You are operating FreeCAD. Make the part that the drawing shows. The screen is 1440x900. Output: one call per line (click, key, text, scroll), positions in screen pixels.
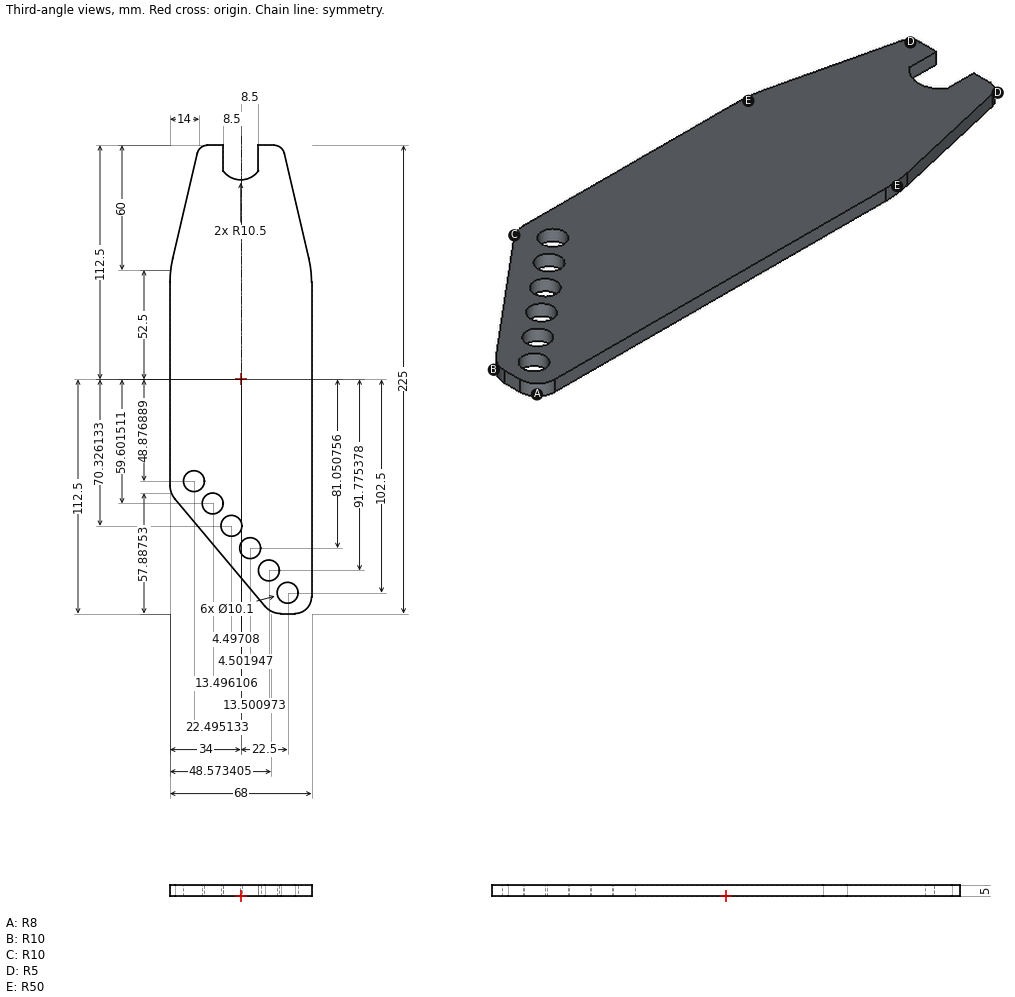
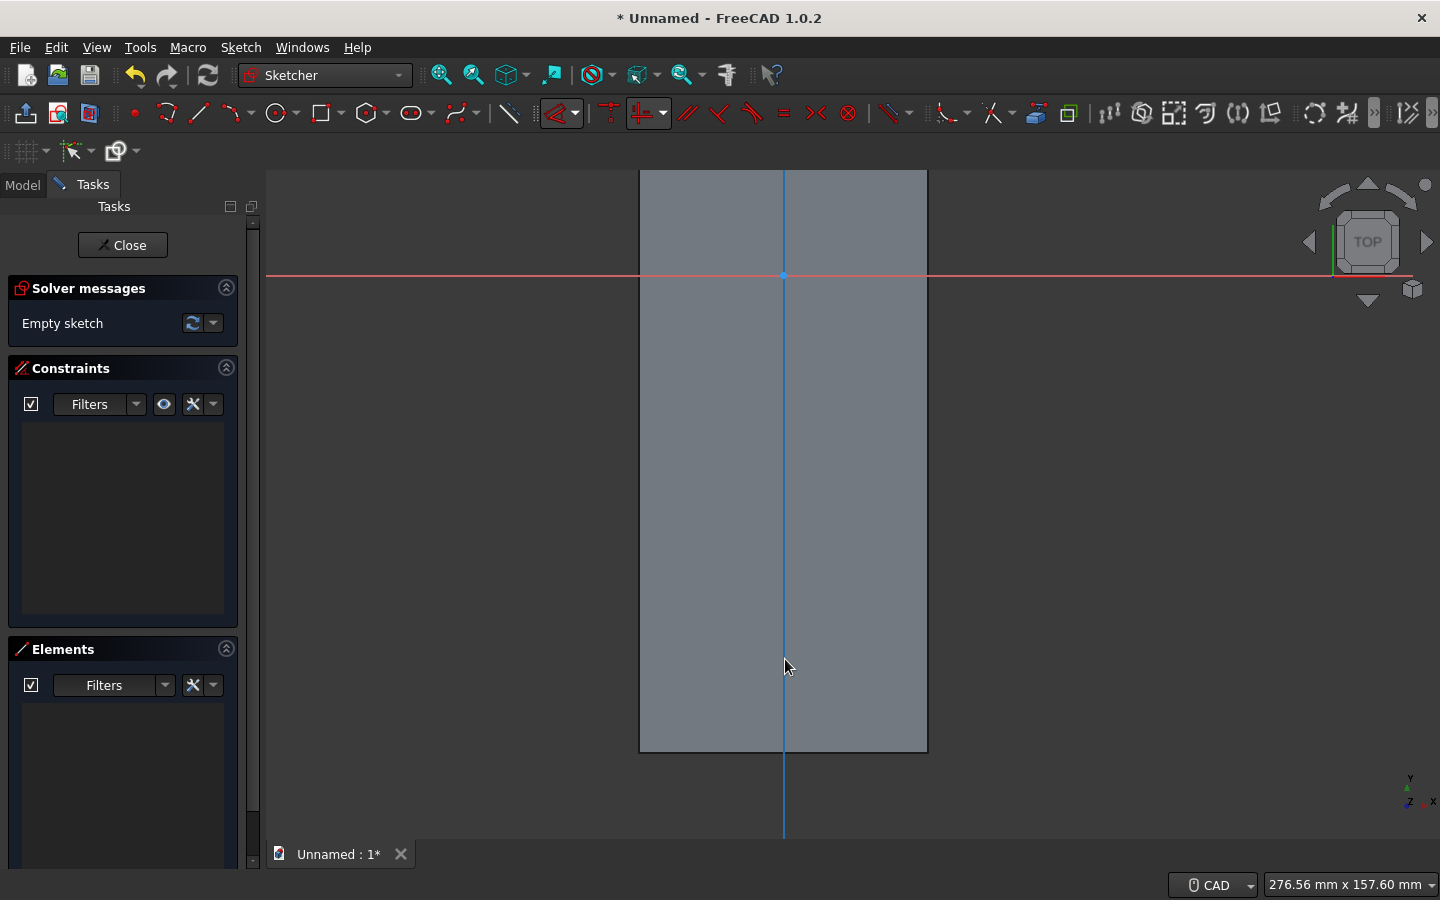
key(g)
key(c)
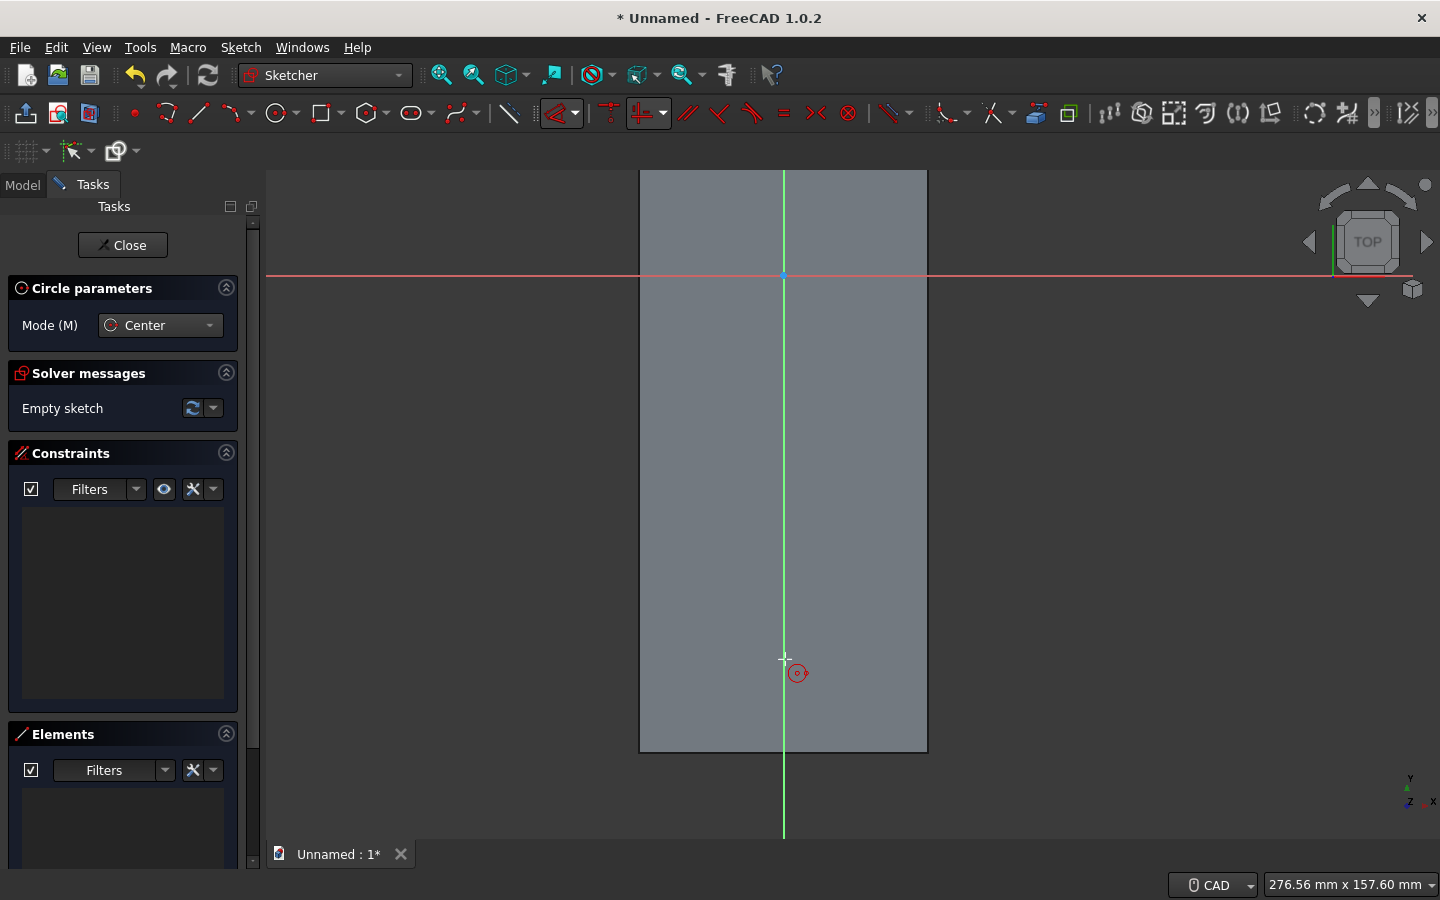
click(879, 711)
click(894, 696)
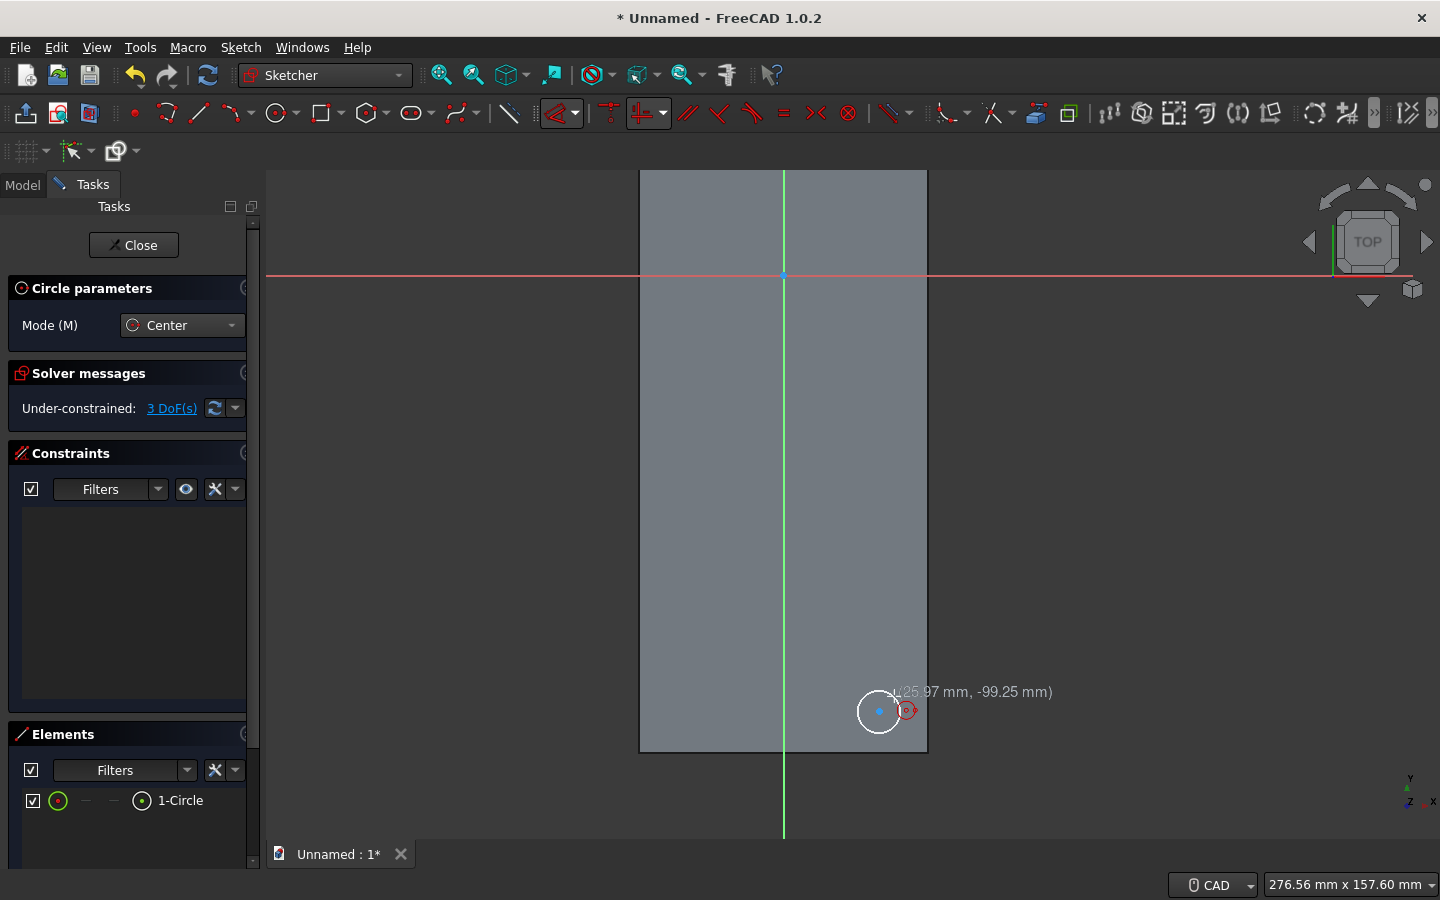
click(841, 665)
click(856, 650)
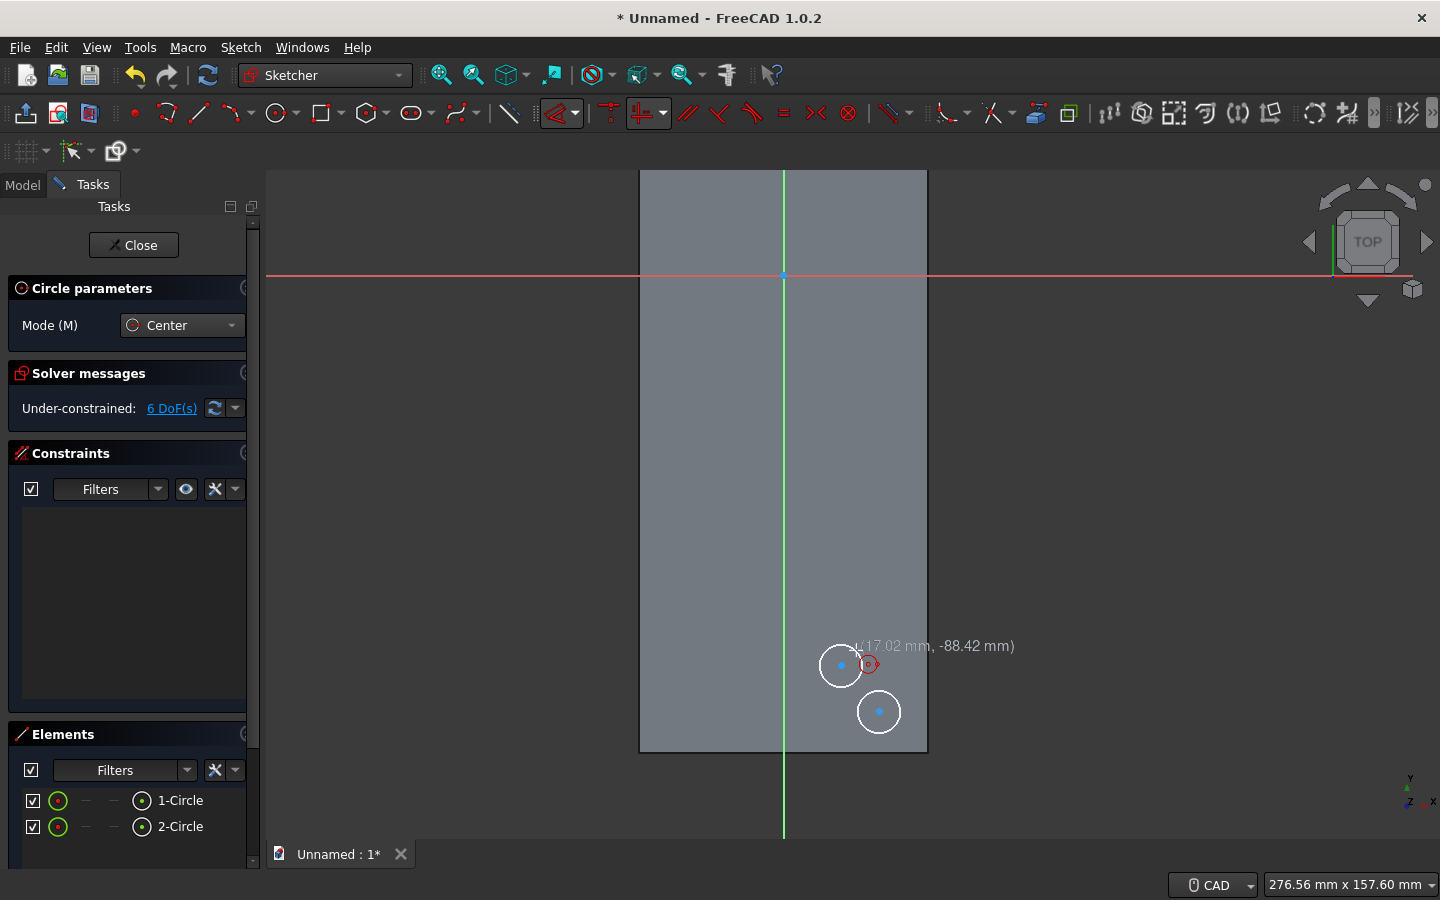
click(803, 620)
click(818, 605)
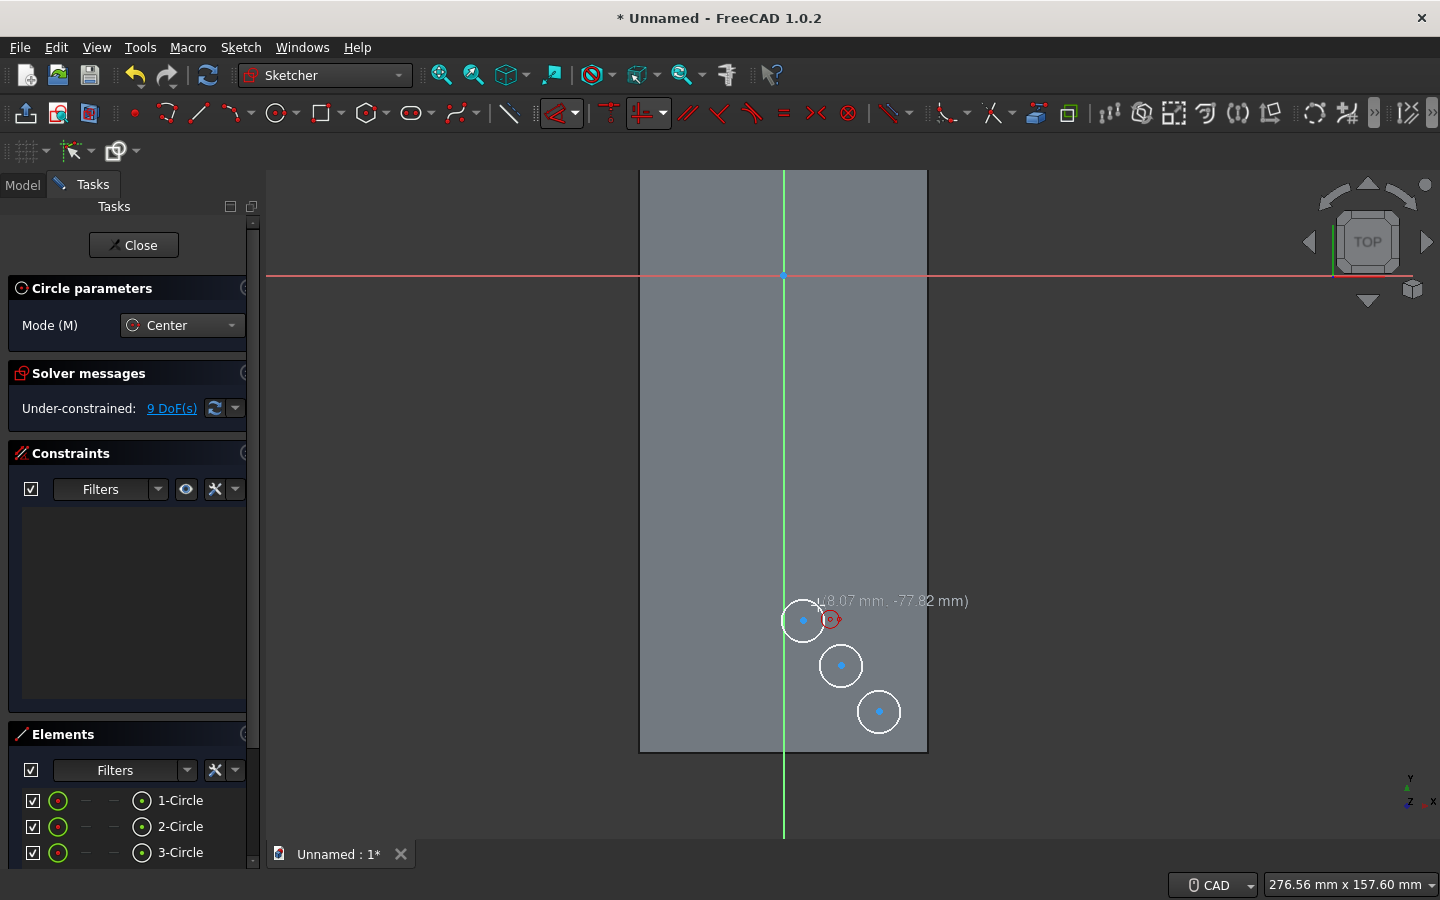
click(765, 574)
click(749, 559)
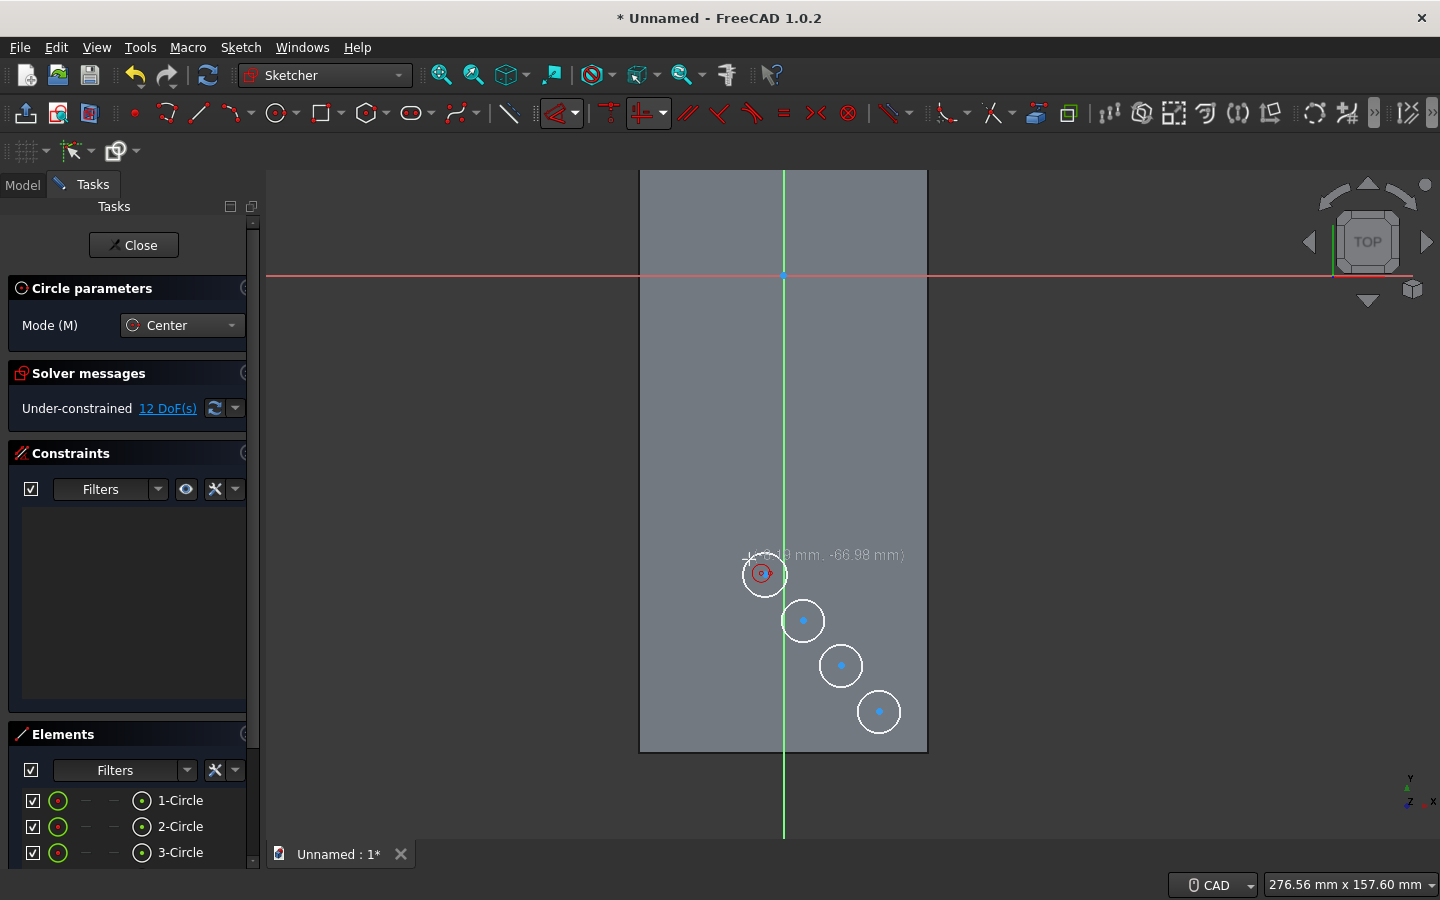
click(726, 529)
click(742, 514)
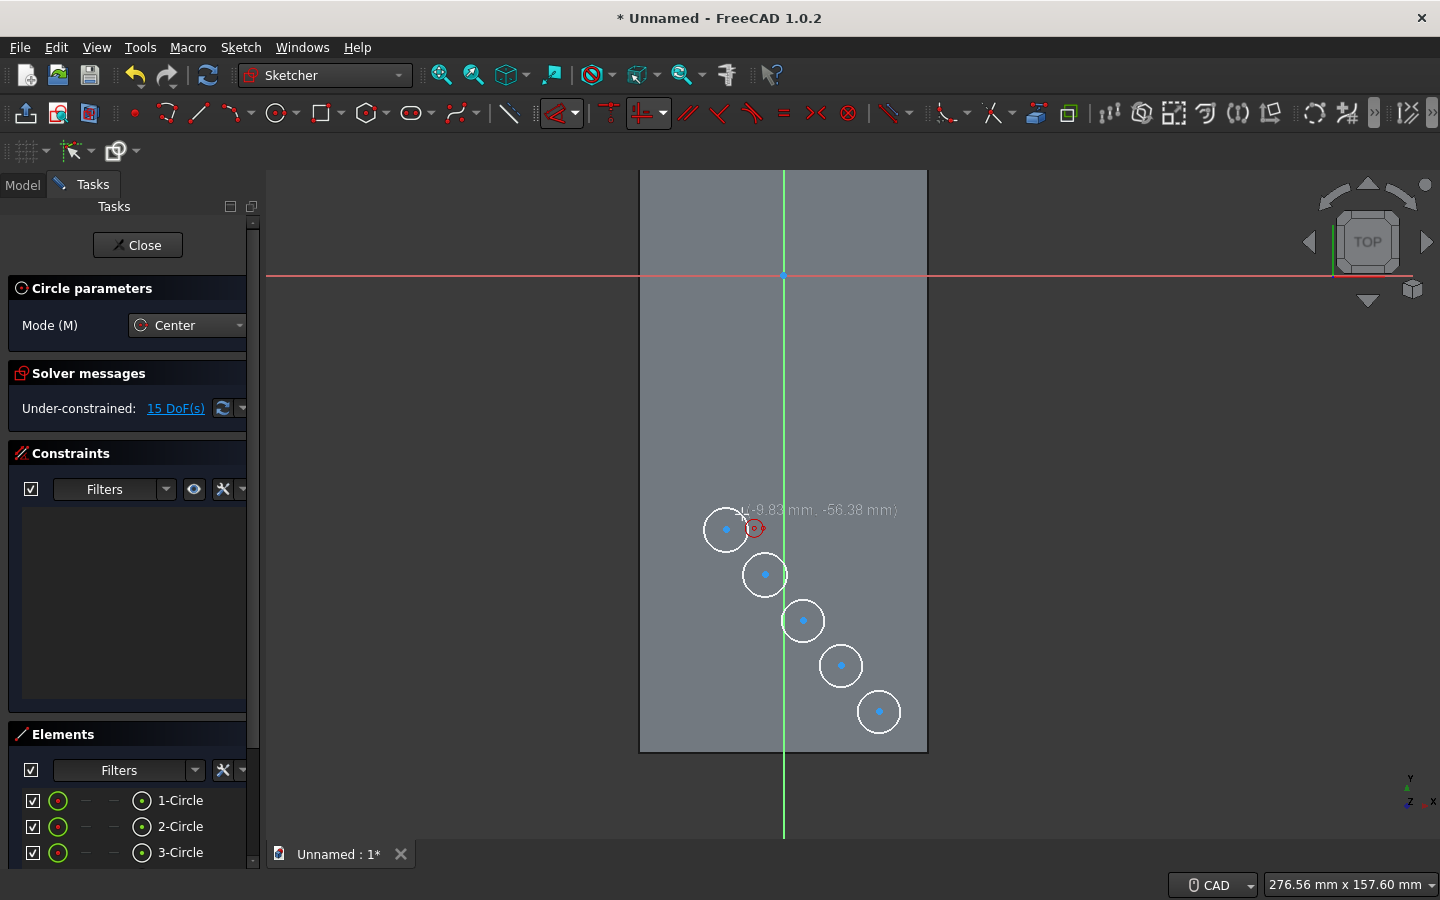
click(688, 483)
click(703, 468)
key(Escape)